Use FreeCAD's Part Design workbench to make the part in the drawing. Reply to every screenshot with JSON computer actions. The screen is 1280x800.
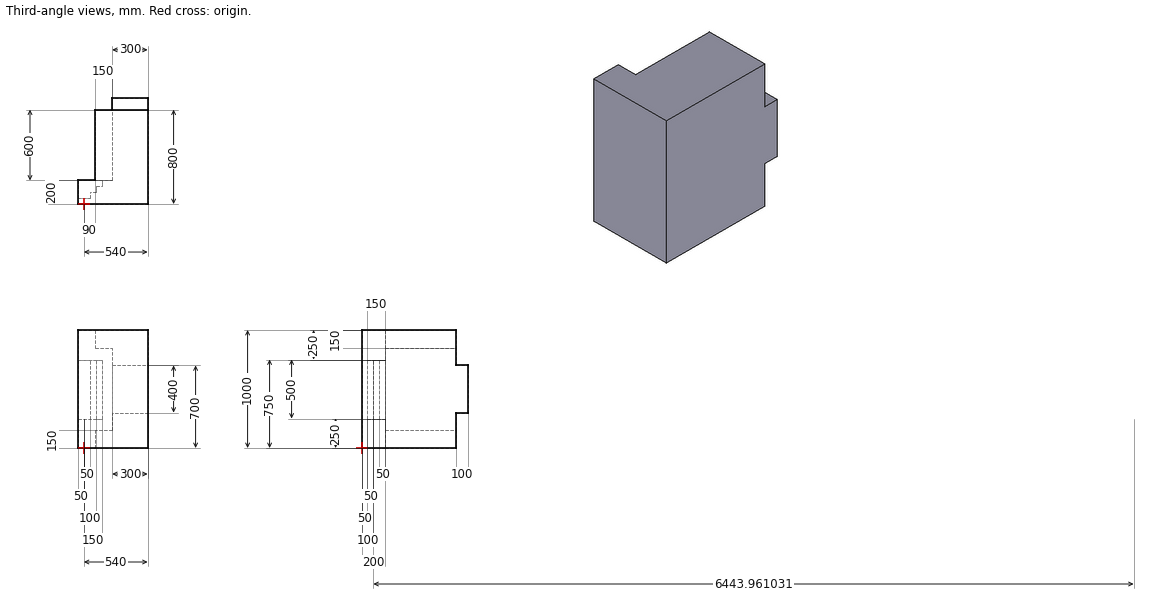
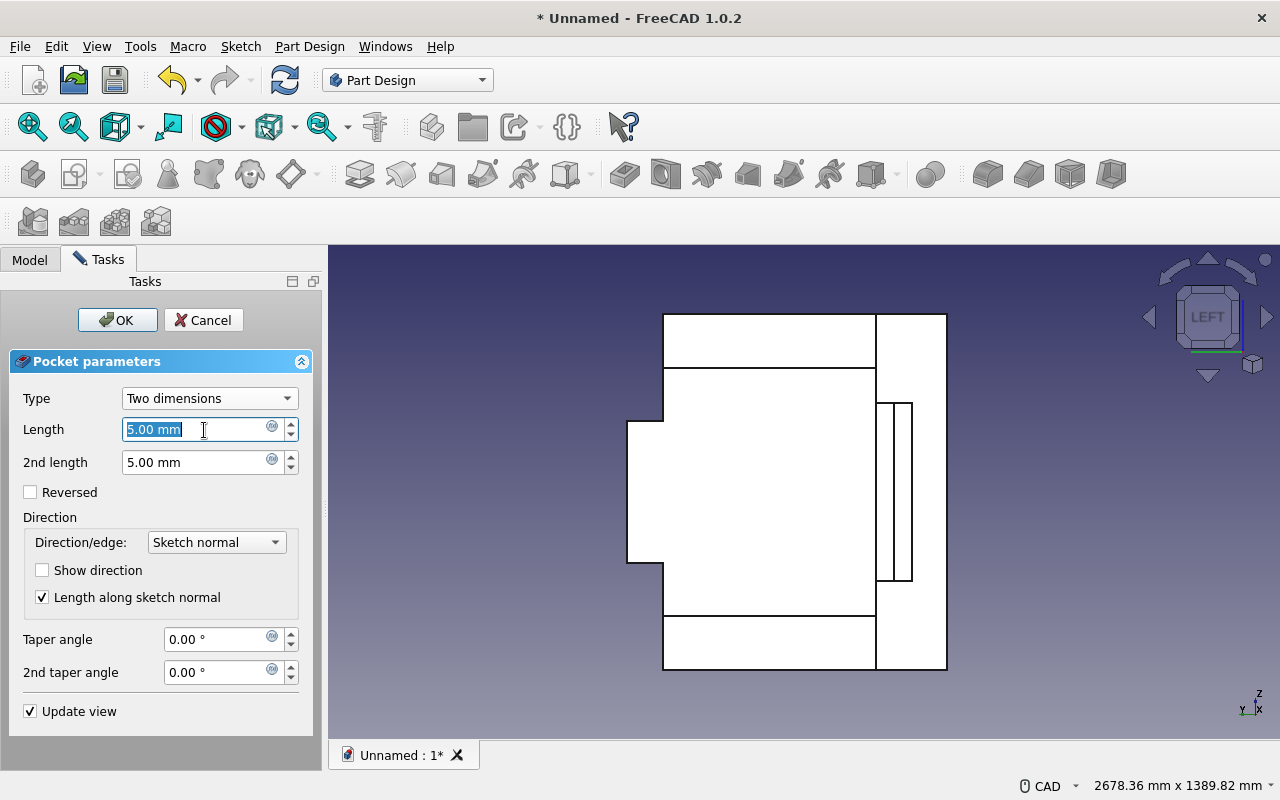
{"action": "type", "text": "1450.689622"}
{"action": "key", "text": "Tab"}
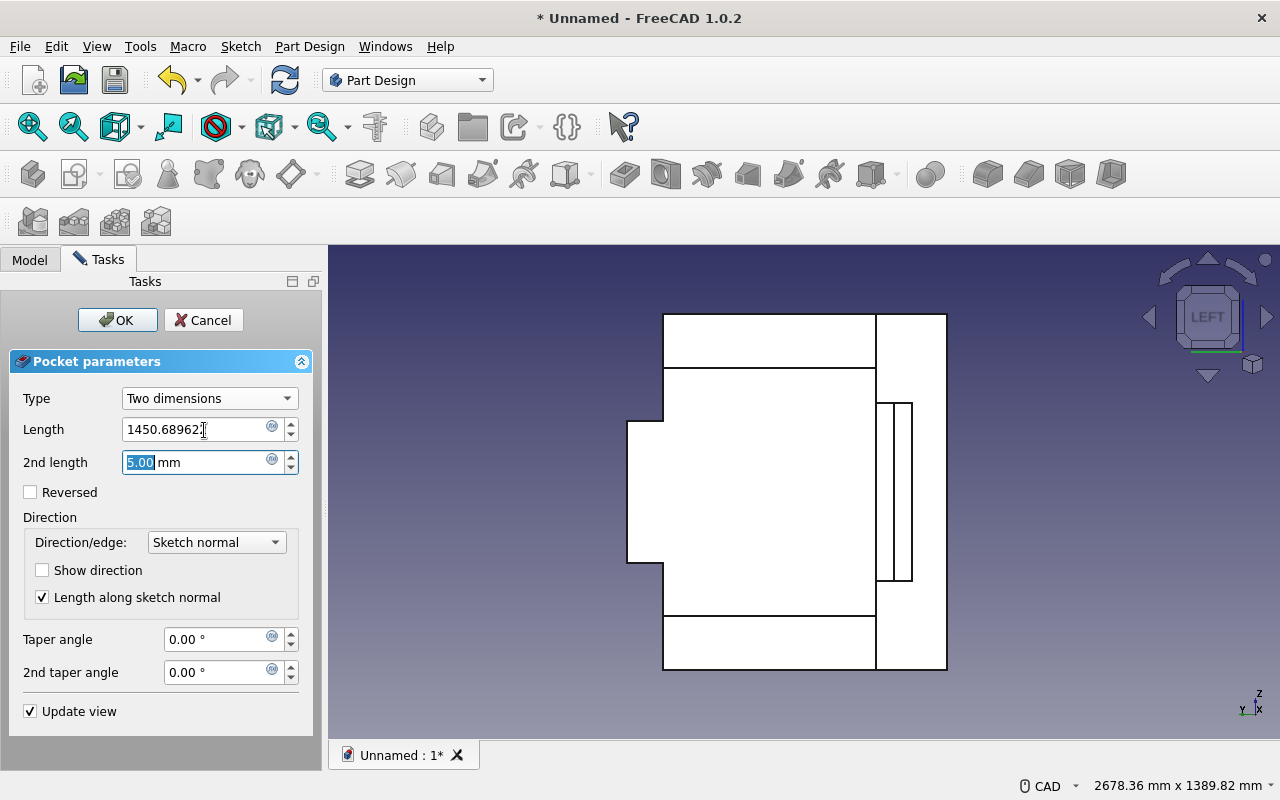
{"action": "type", "text": "100"}
{"action": "key", "text": "Tab"}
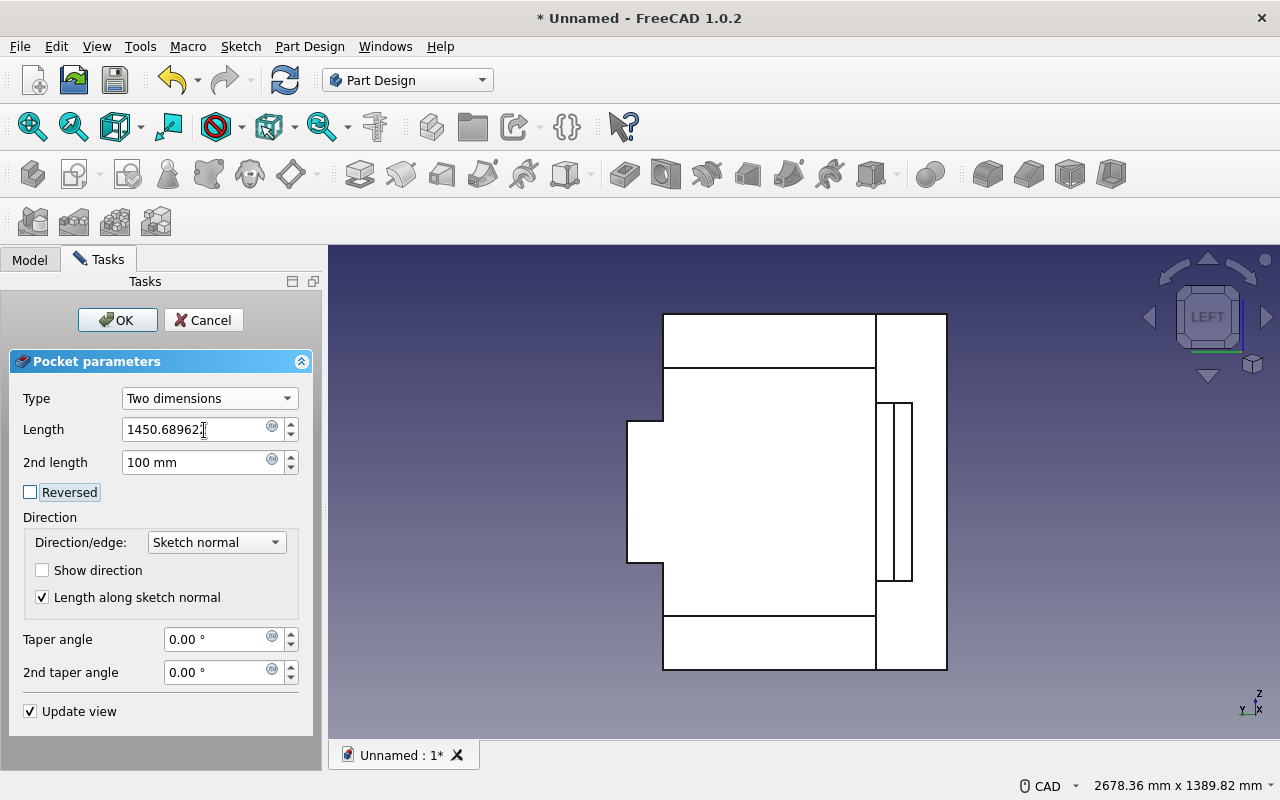
{"action": "left_click", "coordinate": [118, 320]}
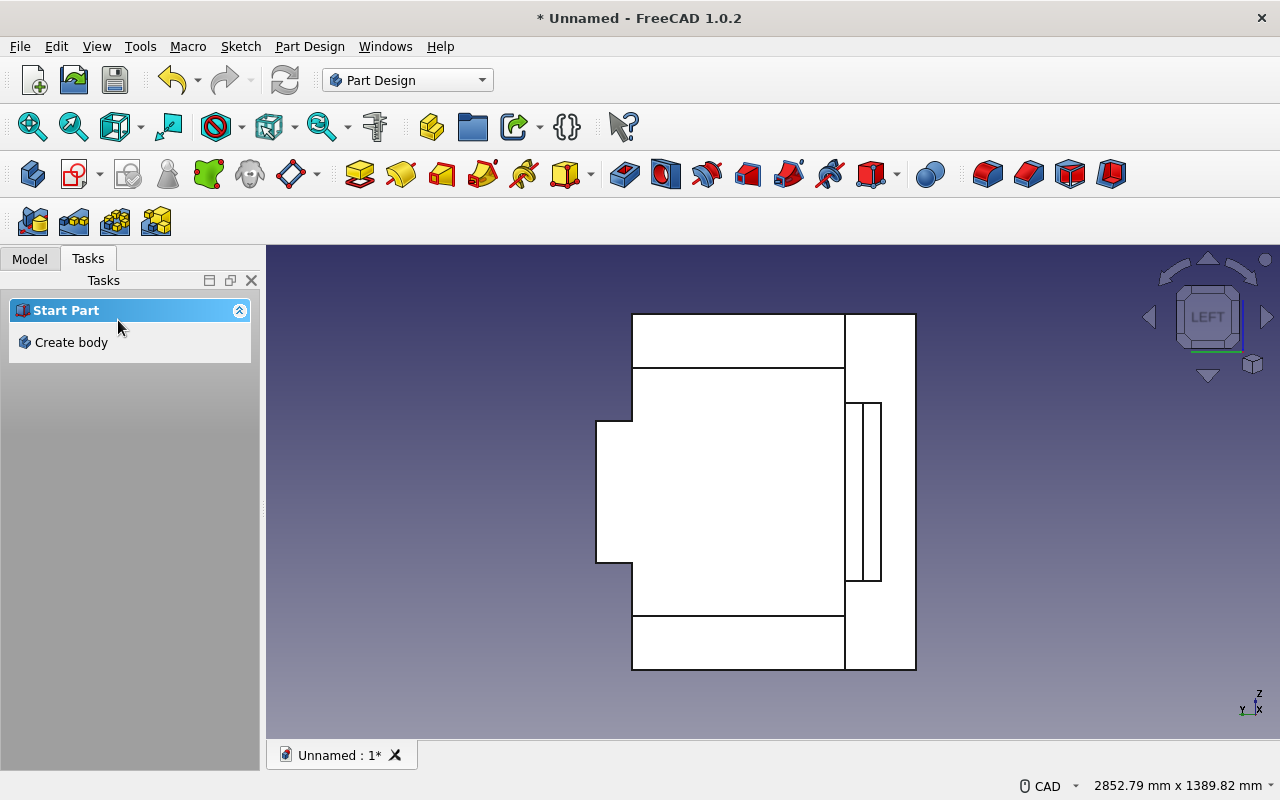
{"action": "left_click", "coordinate": [881, 339]}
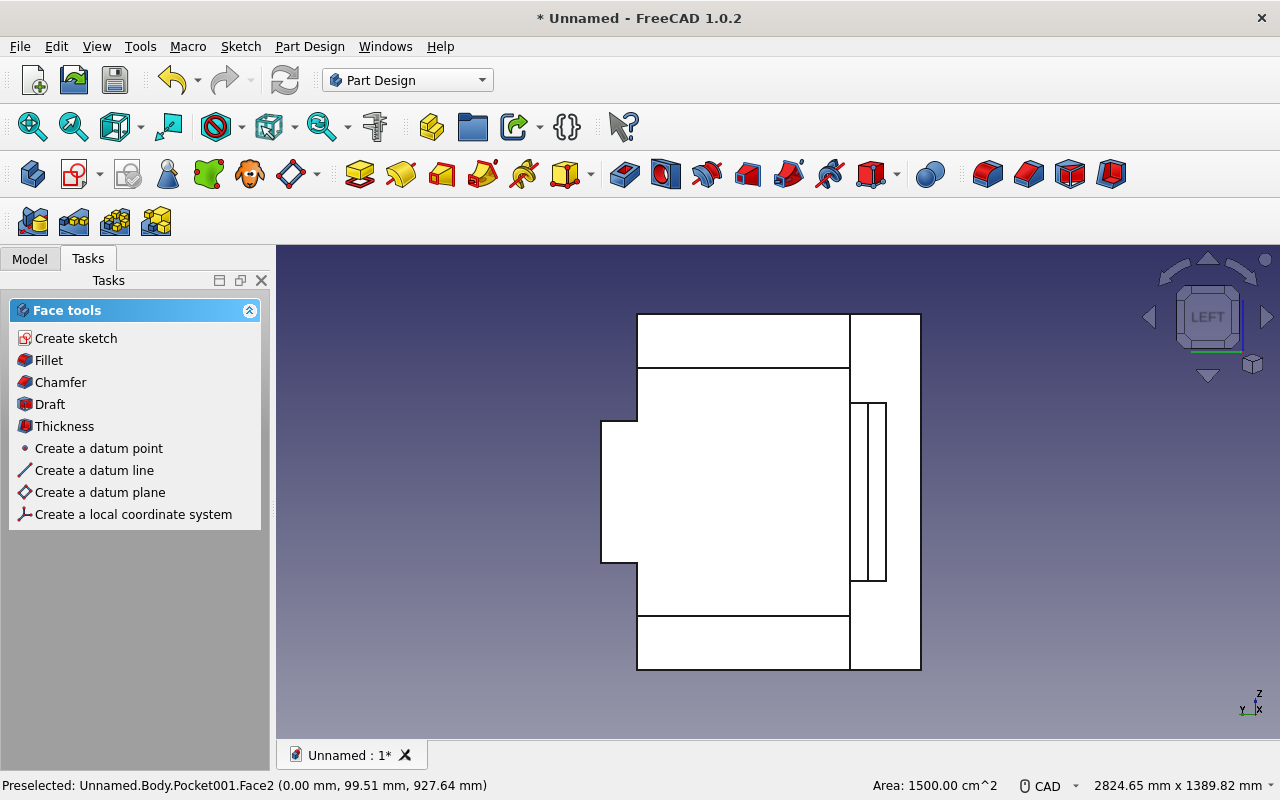
{"action": "left_click", "coordinate": [74, 174]}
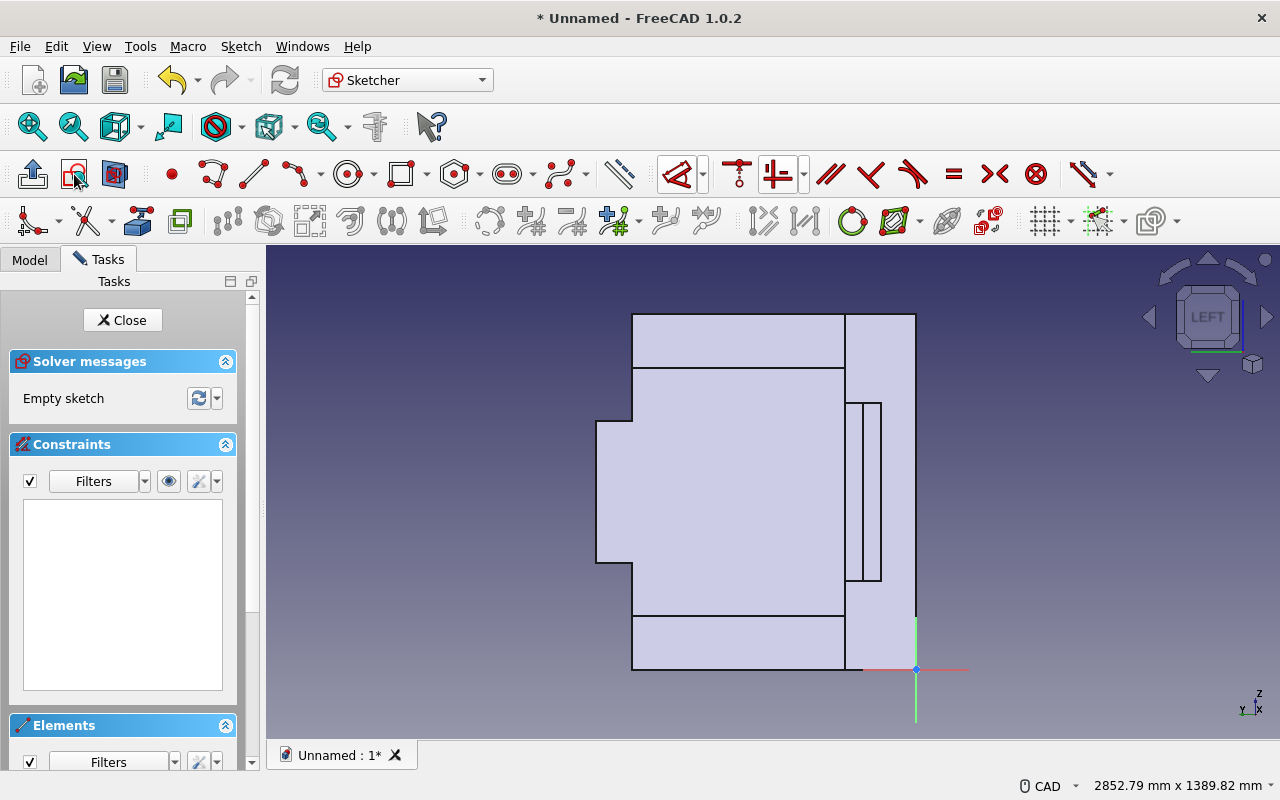
{"action": "left_click", "coordinate": [400, 174]}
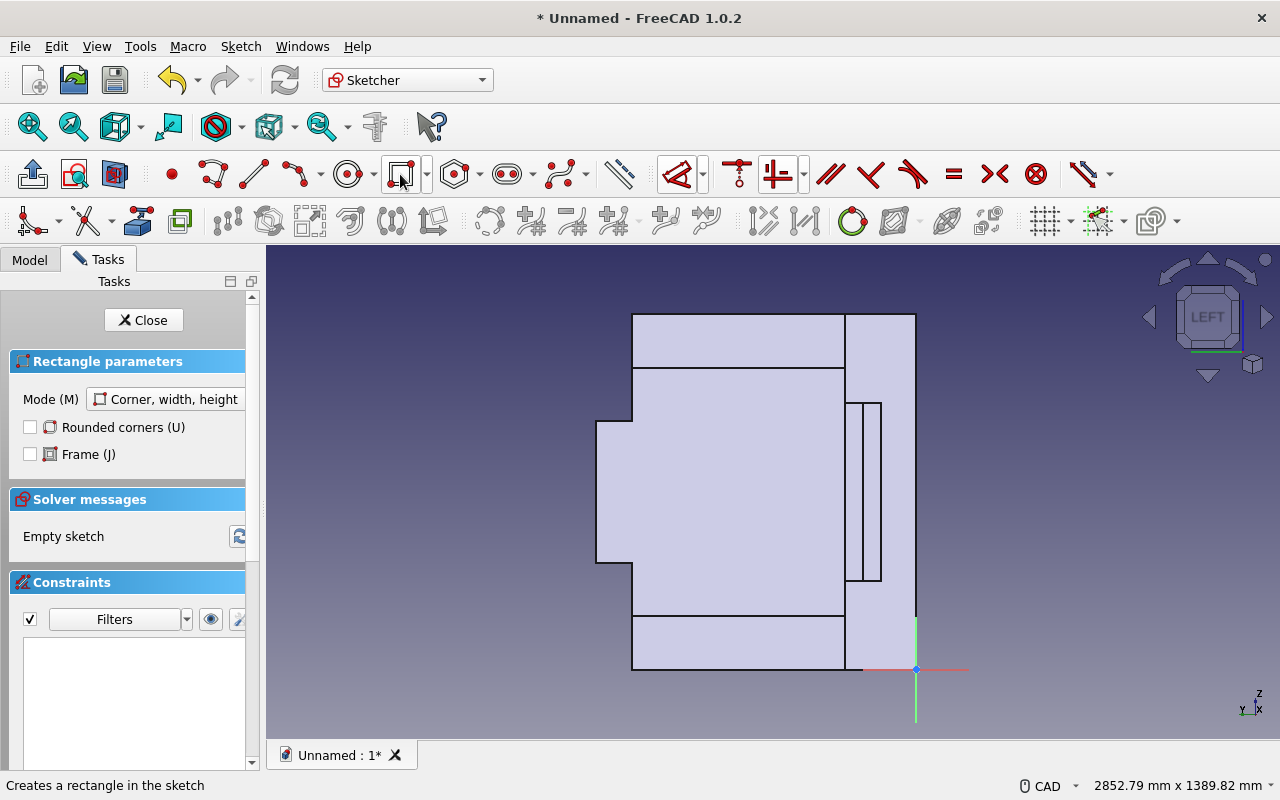
{"action": "left_click", "coordinate": [881, 403]}
{"action": "left_click", "coordinate": [899, 581]}
{"action": "key", "text": "Escape"}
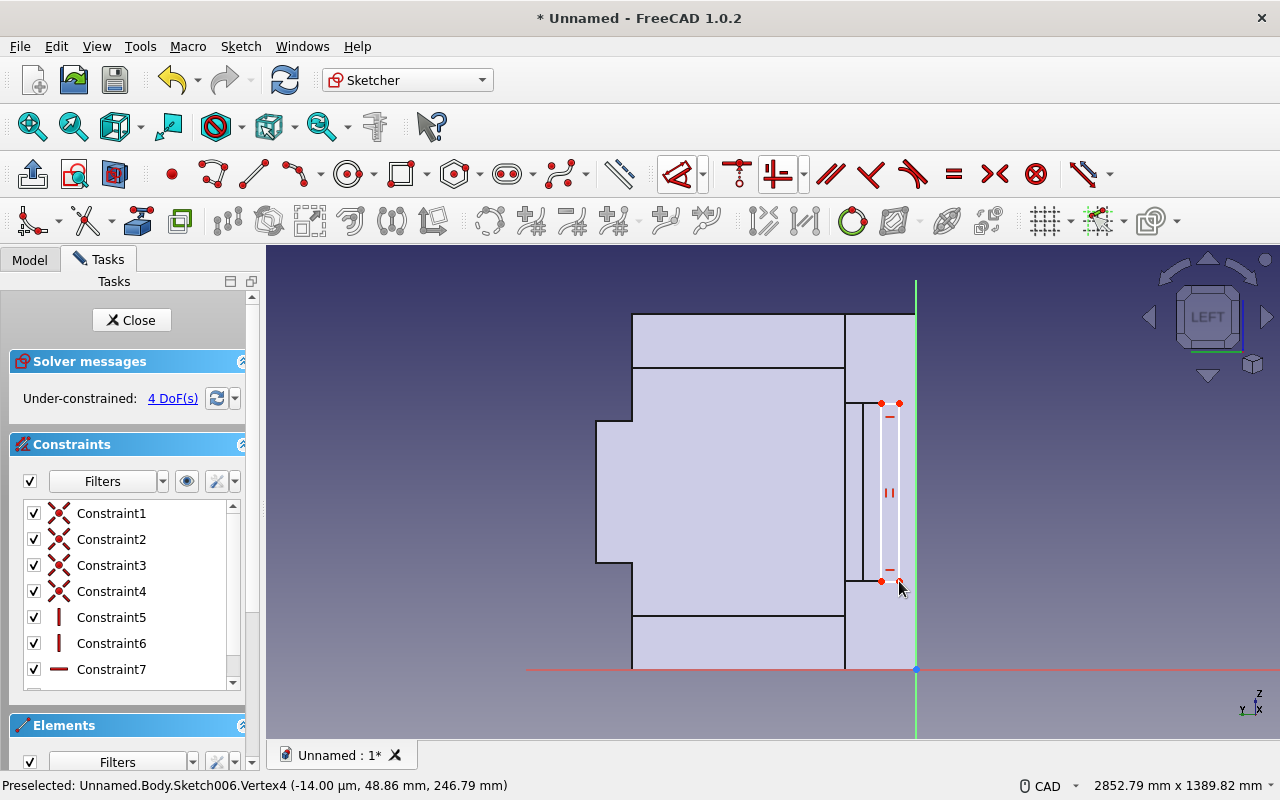
{"action": "scroll", "coordinate": [890, 582], "scroll_direction": "up", "scroll_amount": 5}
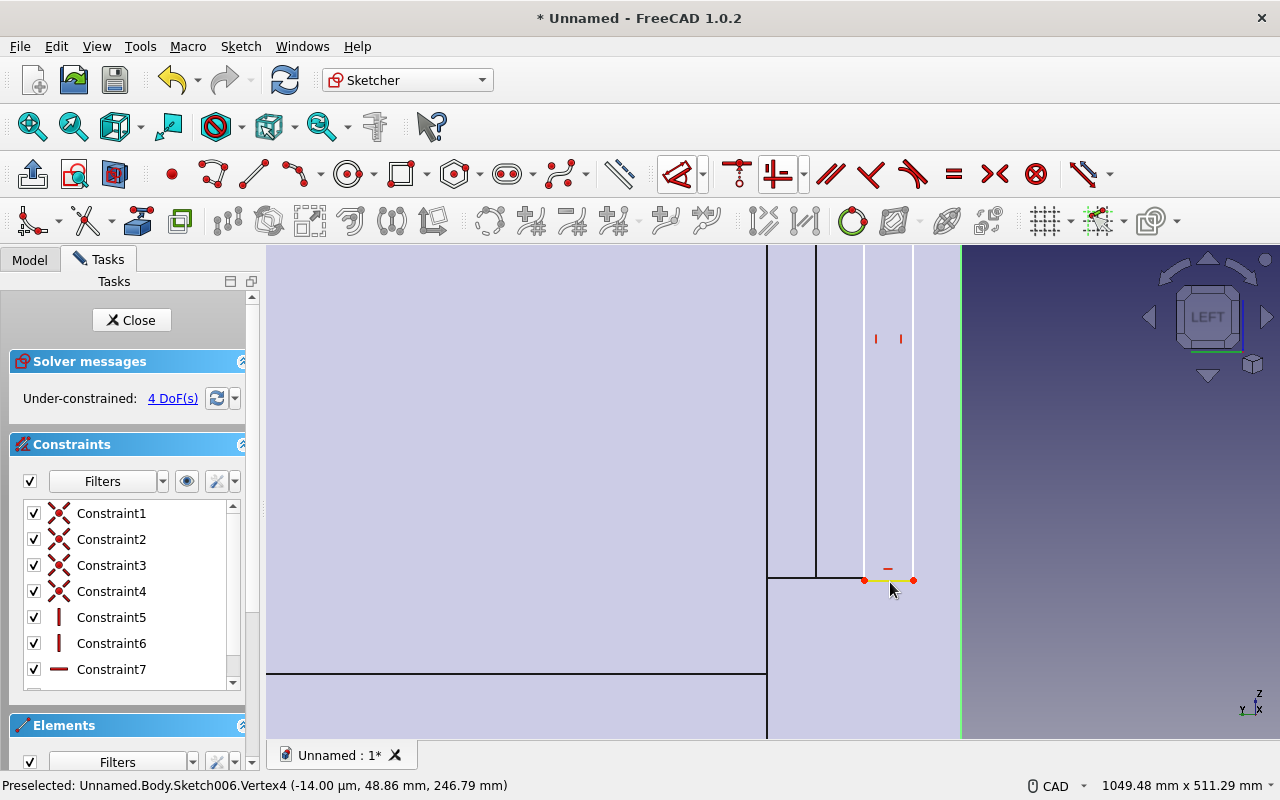
{"action": "left_click", "coordinate": [889, 581]}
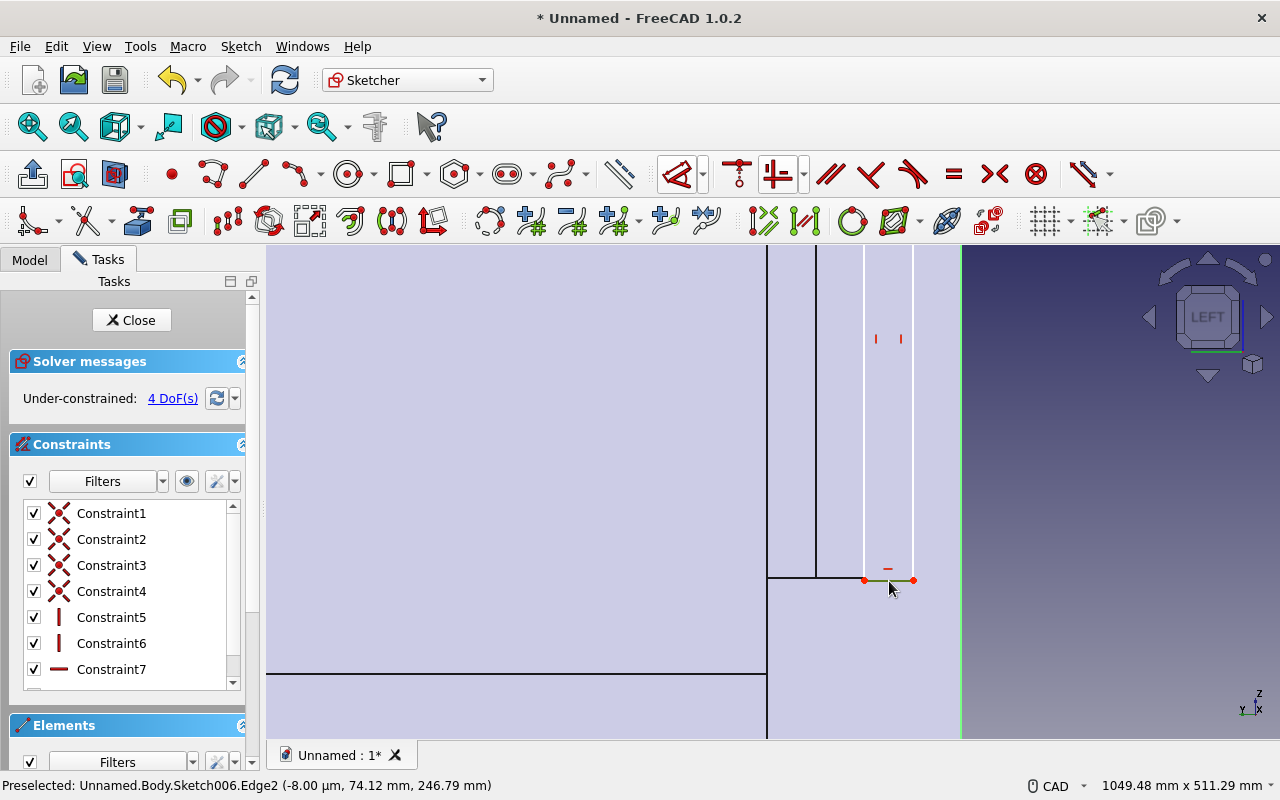
{"action": "left_click", "coordinate": [702, 174]}